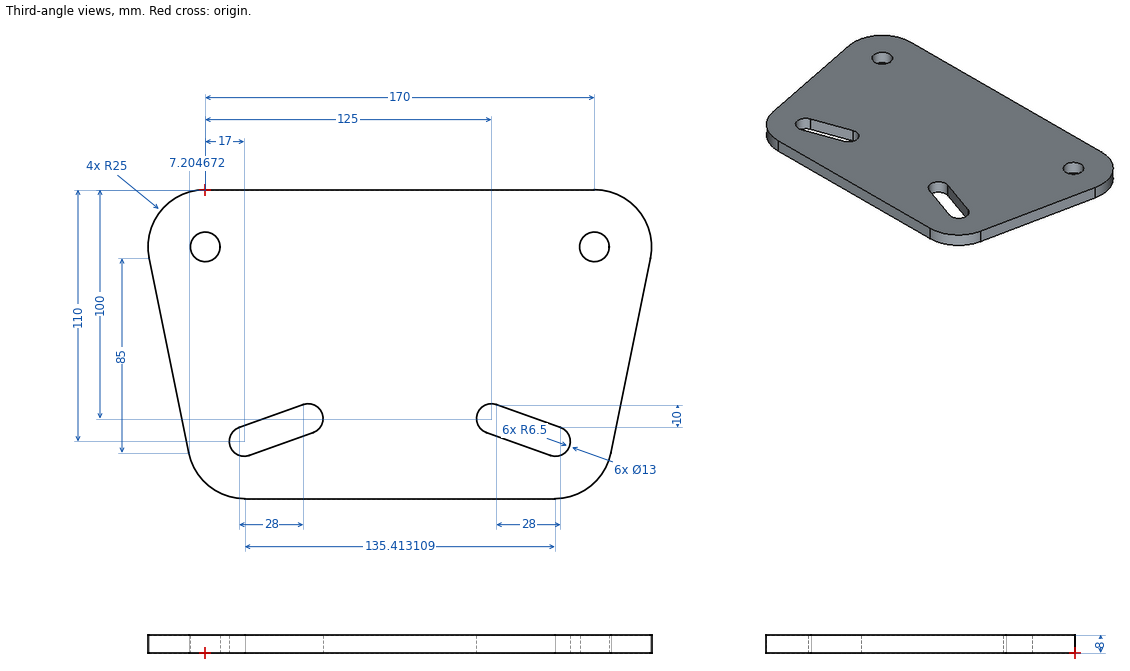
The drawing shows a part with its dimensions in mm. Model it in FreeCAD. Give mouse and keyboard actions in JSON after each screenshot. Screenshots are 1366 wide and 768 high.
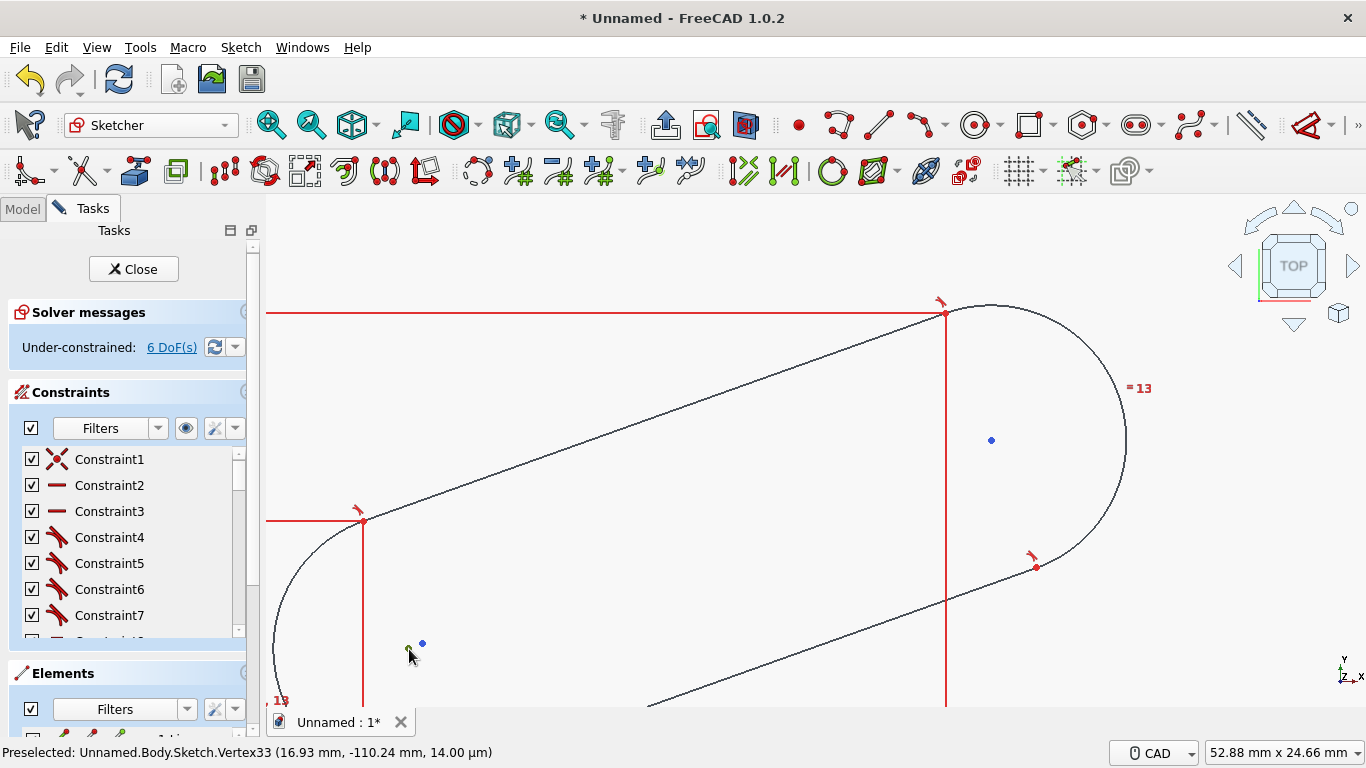
{"action": "key", "text": "l"}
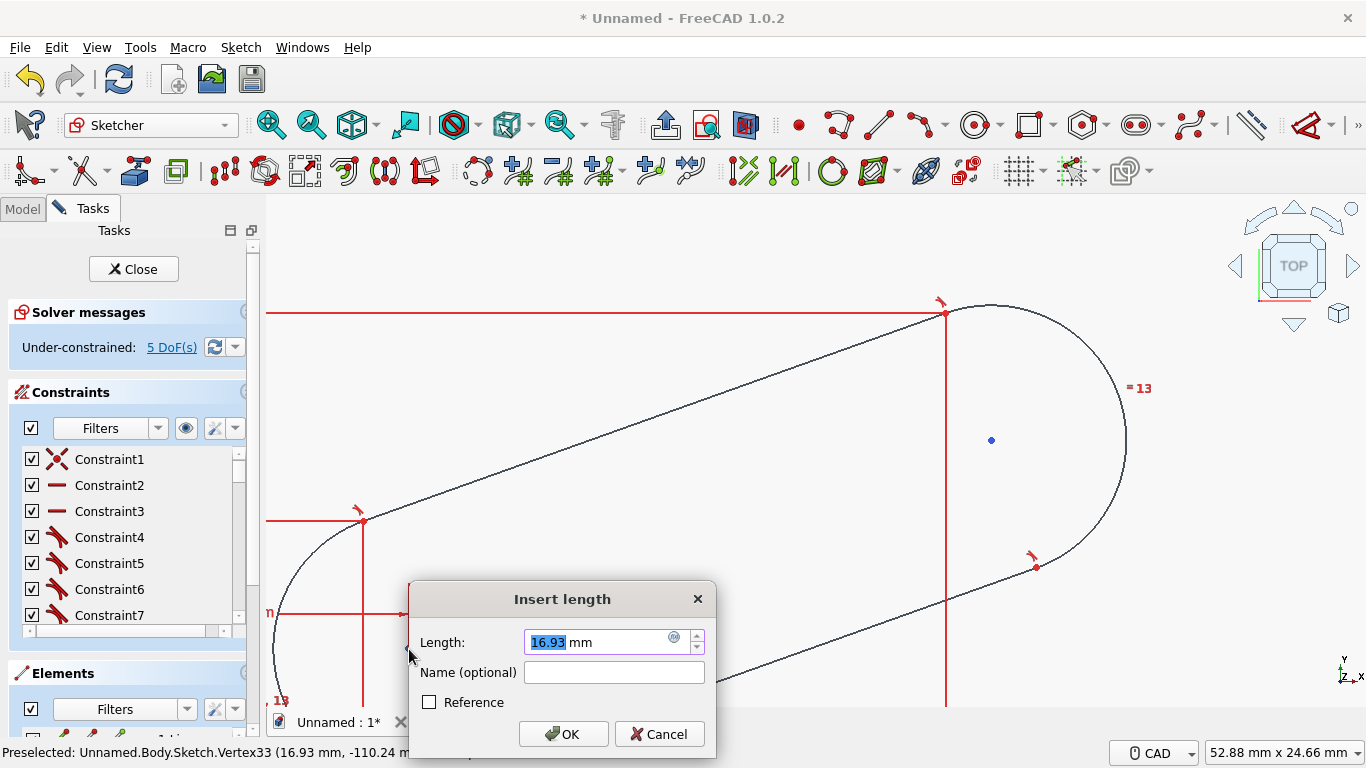
{"action": "type", "text": "17"}
{"action": "key", "text": "Return"}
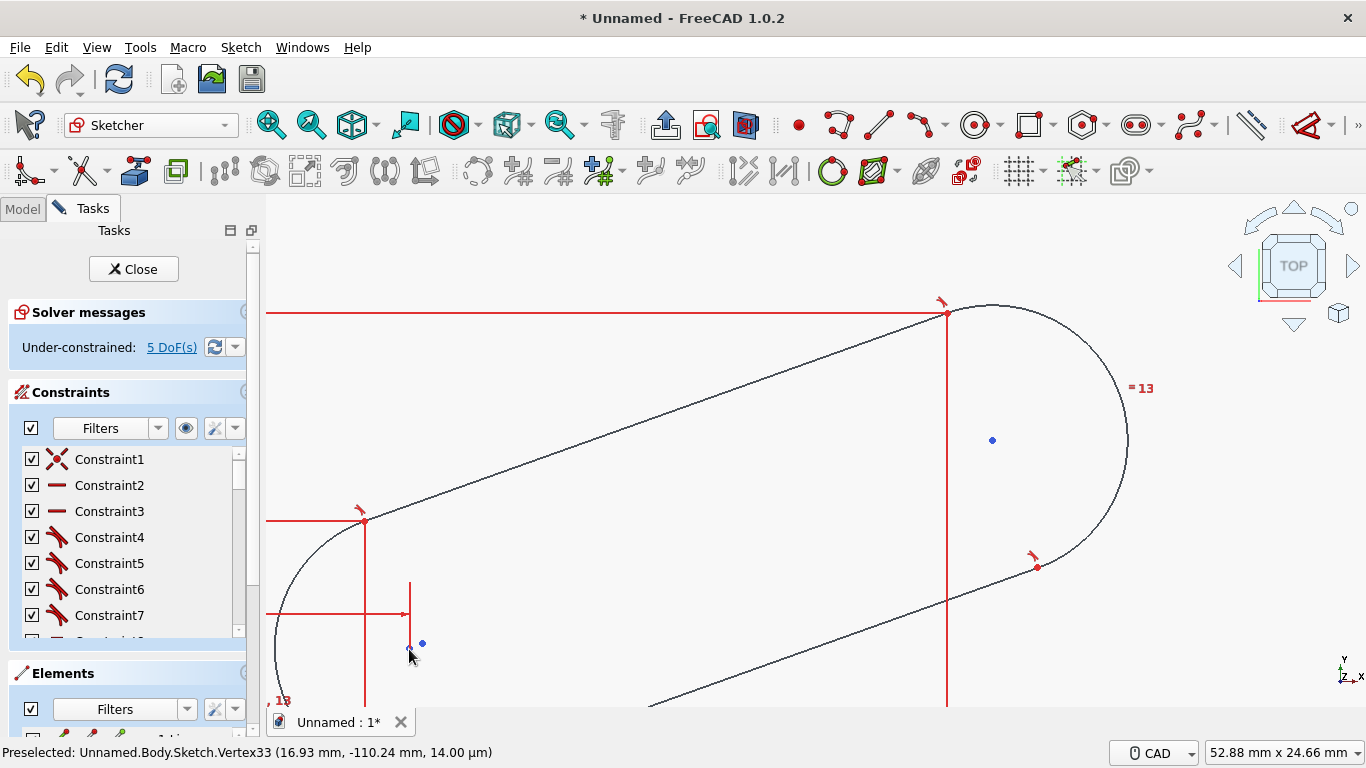
{"action": "scroll", "coordinate": [613, 537], "scroll_direction": "down", "scroll_amount": 11}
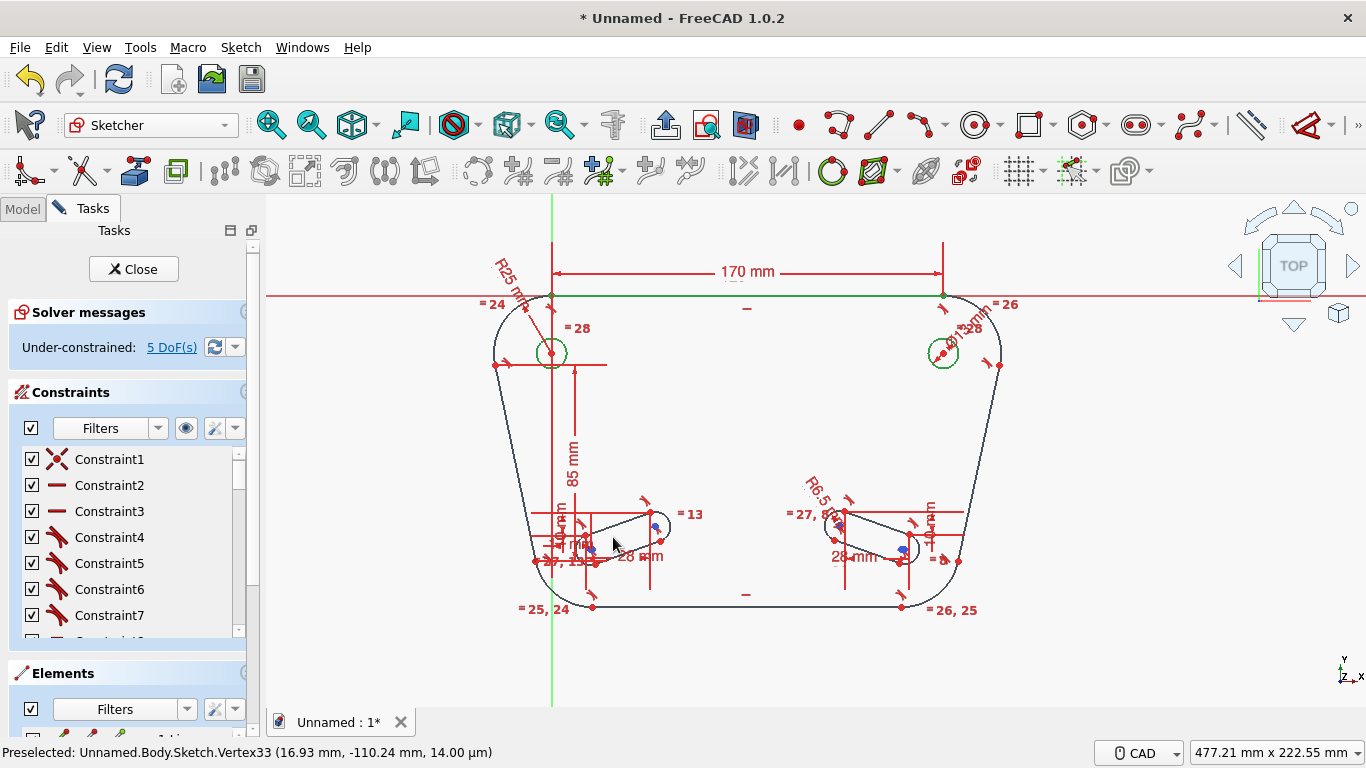
{"action": "left_click", "coordinate": [840, 526]}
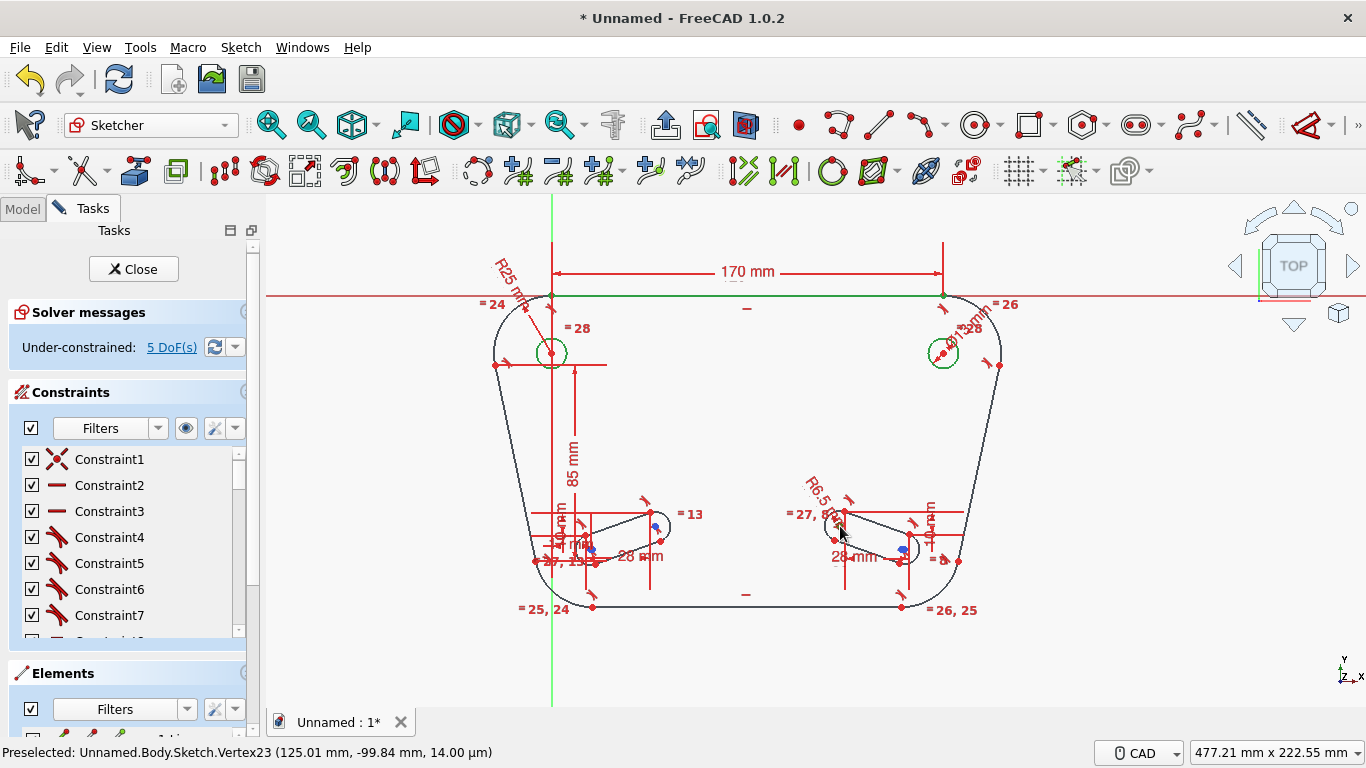
{"action": "left_click", "coordinate": [1334, 126]}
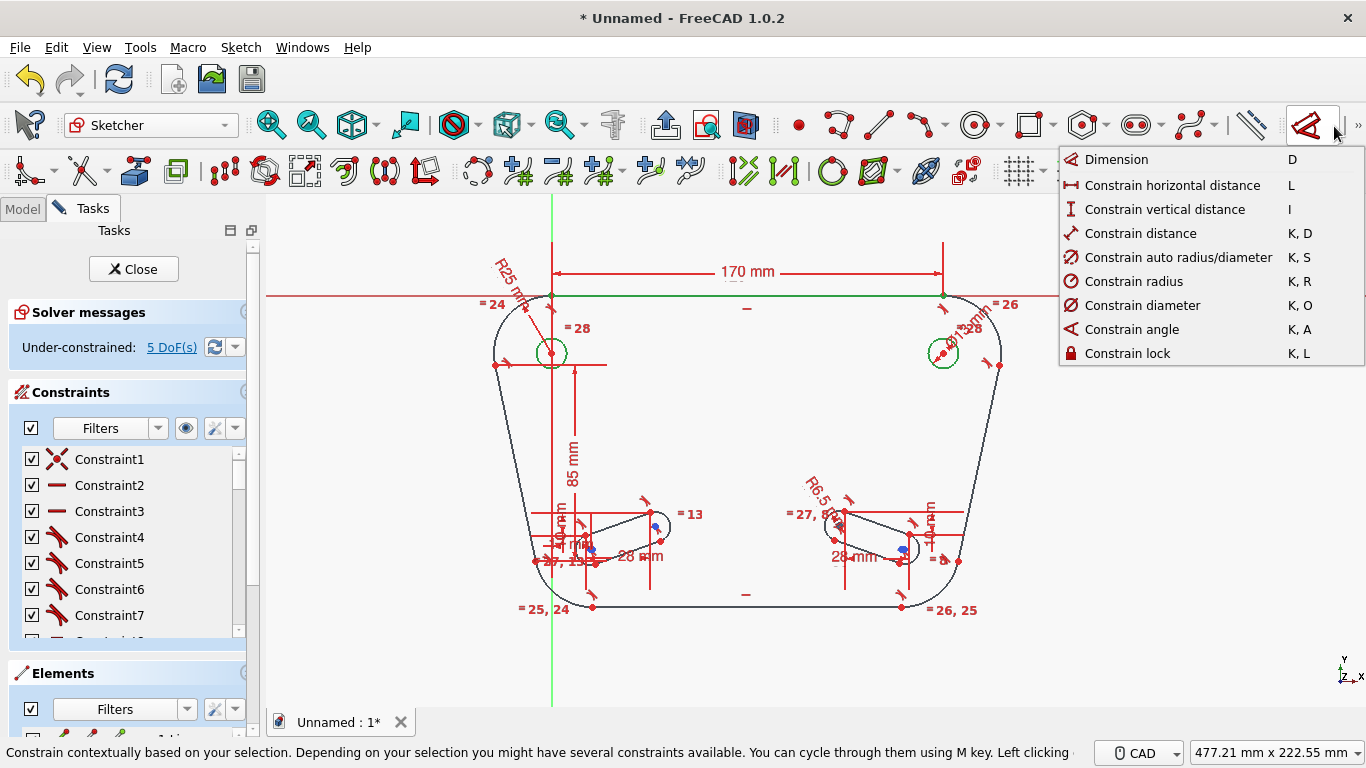
{"action": "left_click", "coordinate": [1212, 185]}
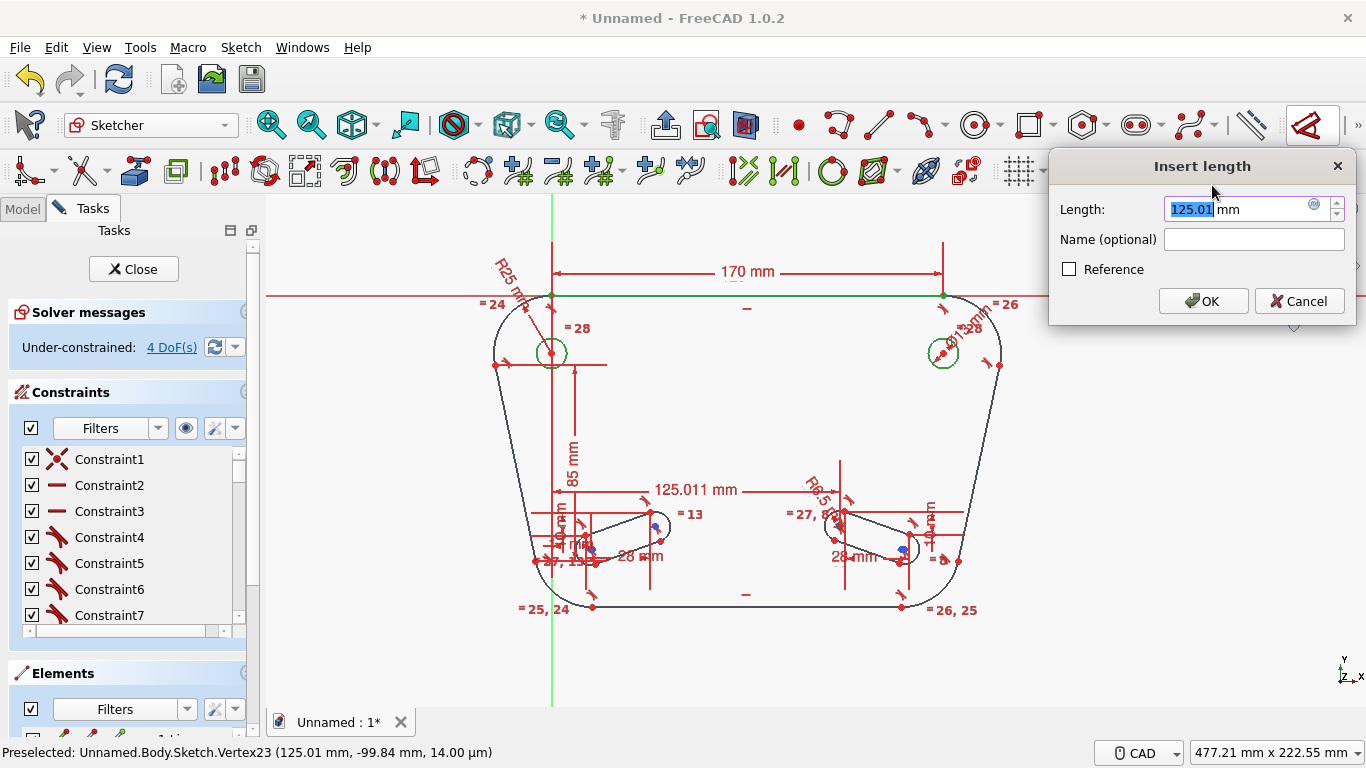
{"action": "type", "text": "125"}
{"action": "key", "text": "Return"}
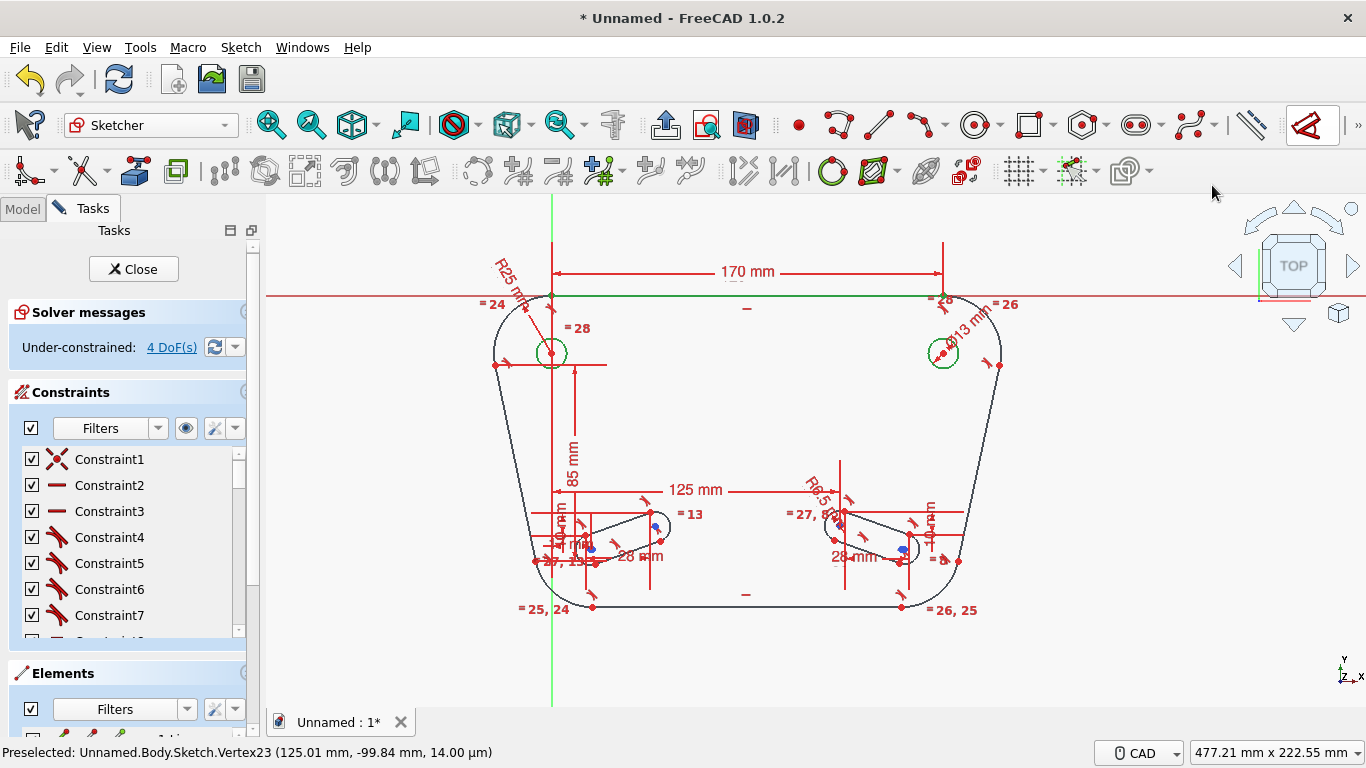
{"action": "left_click", "coordinate": [840, 526]}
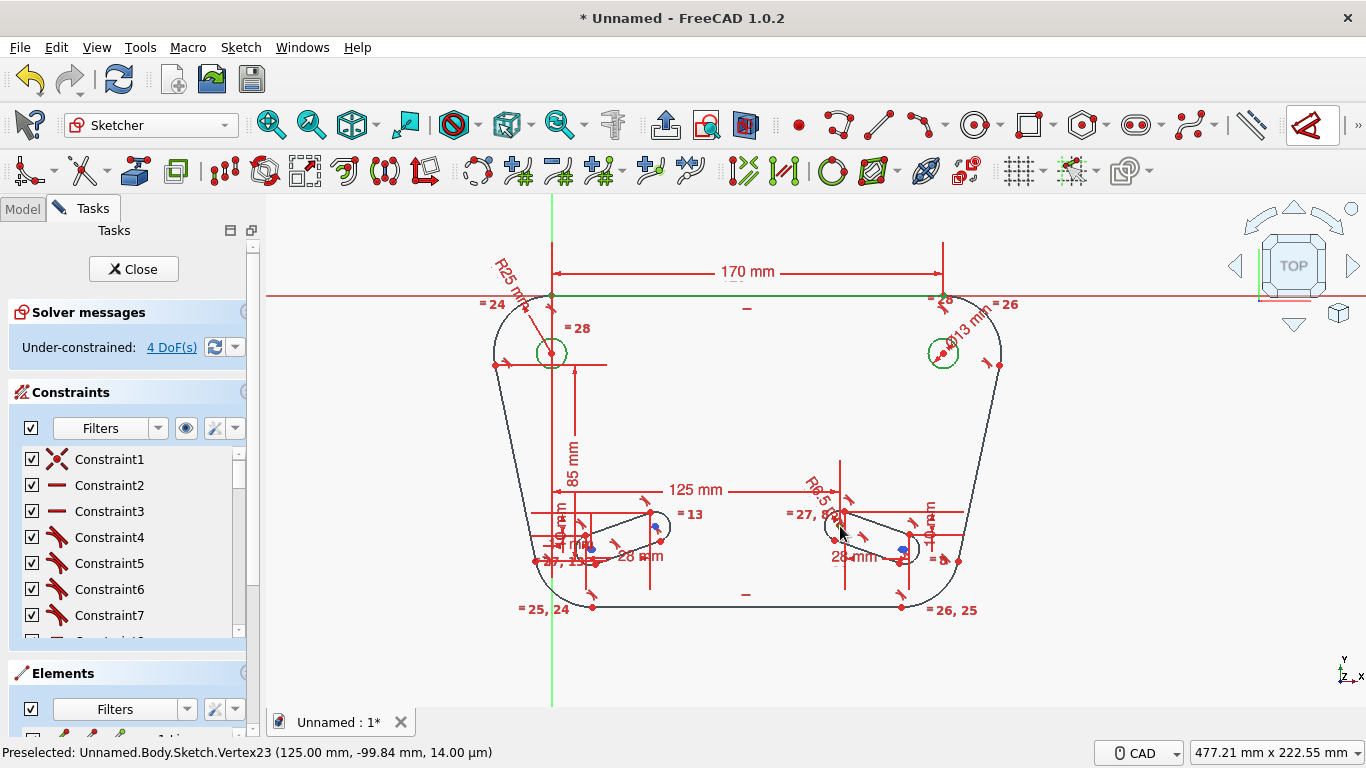
{"action": "left_click", "coordinate": [1334, 126]}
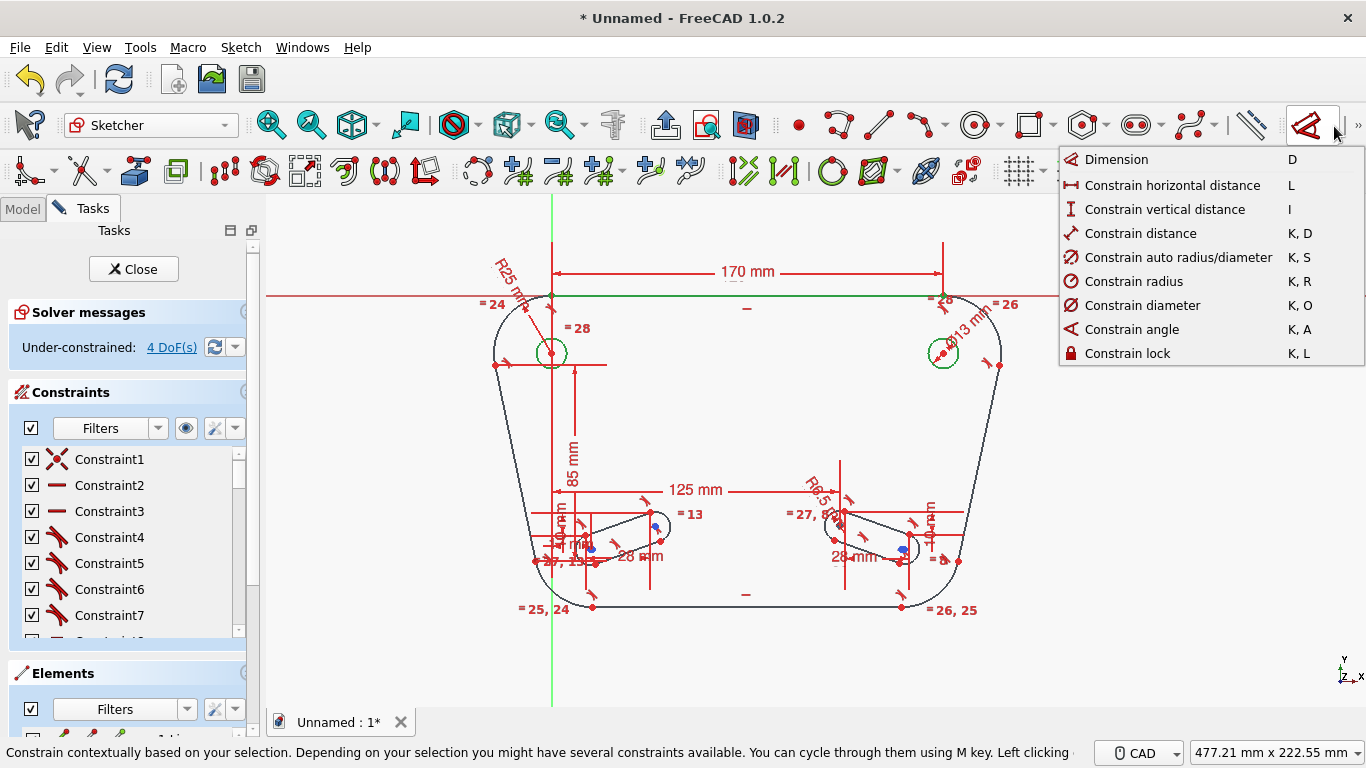
{"action": "left_click", "coordinate": [1212, 209]}